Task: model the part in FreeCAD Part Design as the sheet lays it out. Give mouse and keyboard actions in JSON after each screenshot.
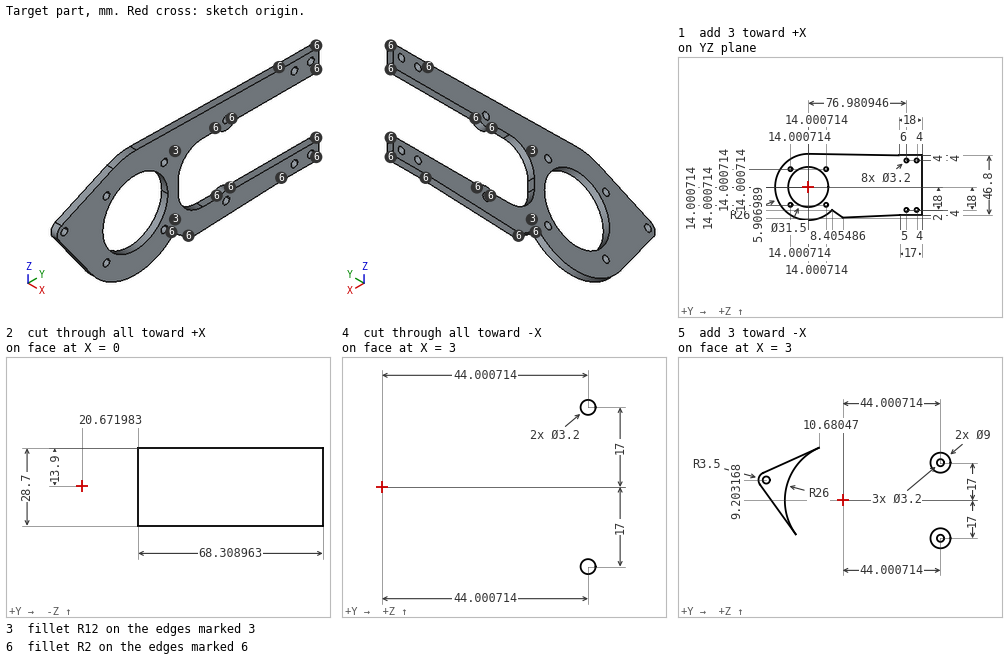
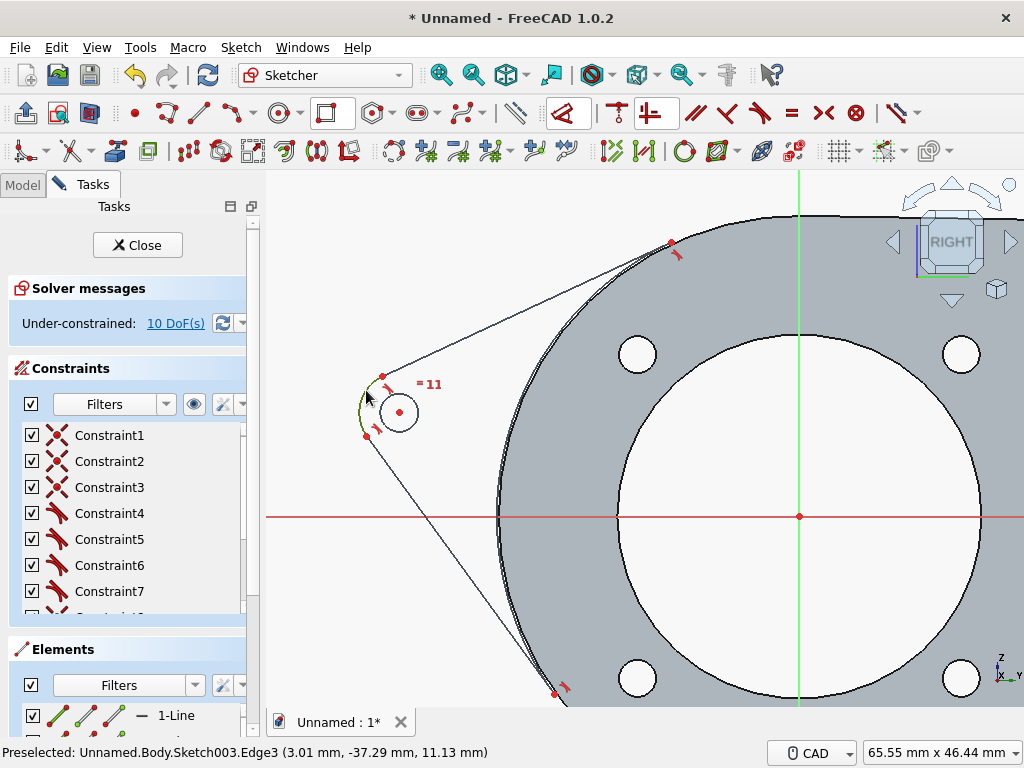
{"action": "left_click", "coordinate": [586, 114]}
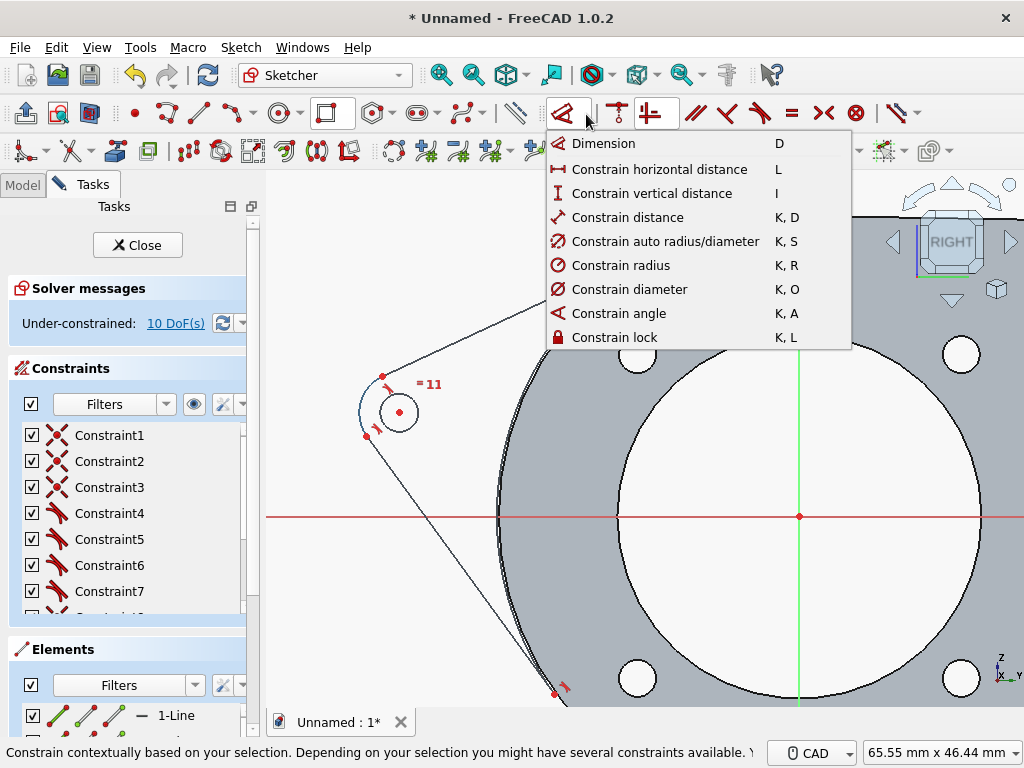
{"action": "left_click", "coordinate": [699, 265]}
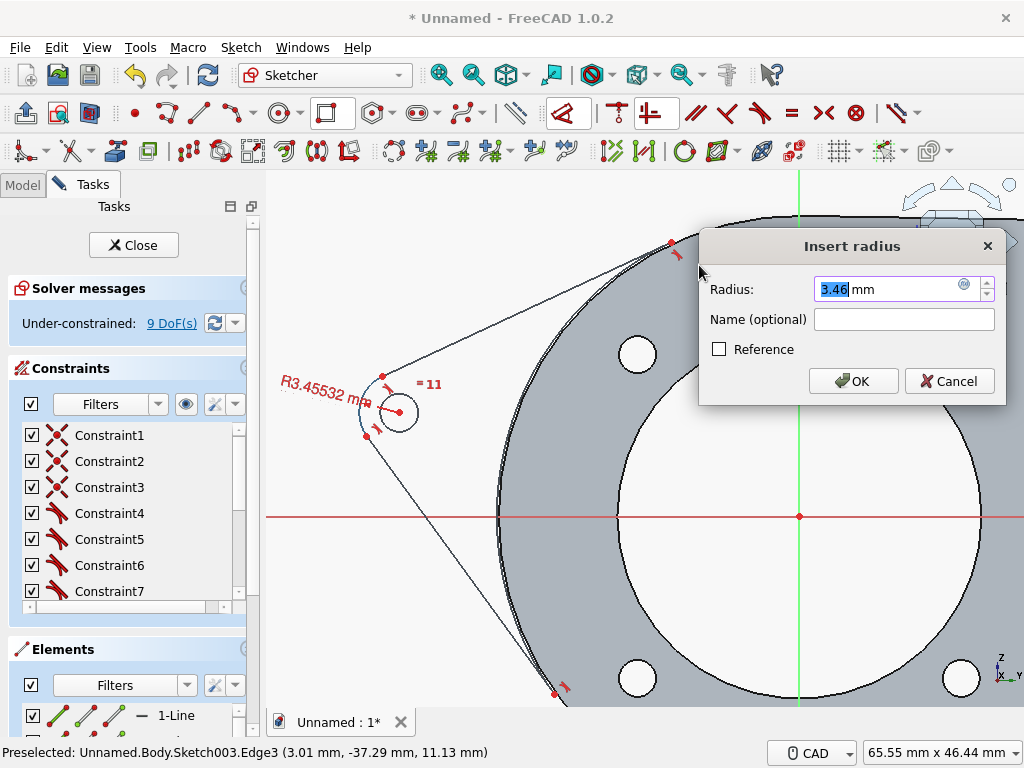
{"action": "type", "text": "3.5"}
{"action": "key", "text": "Return"}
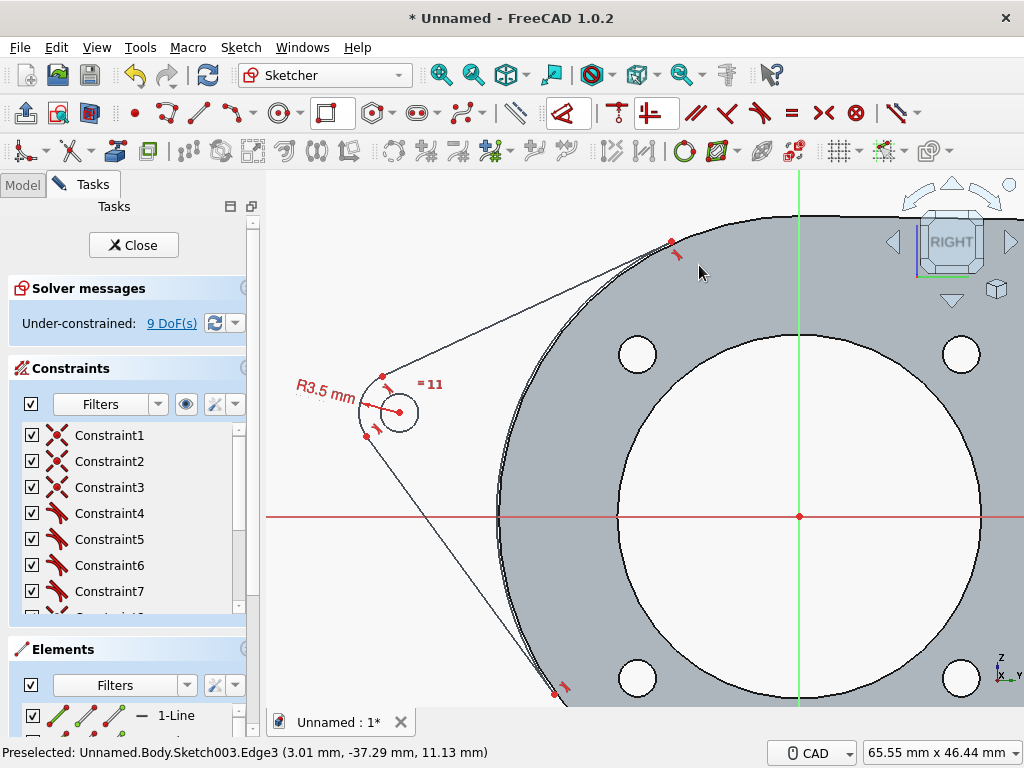
{"action": "left_click", "coordinate": [551, 344]}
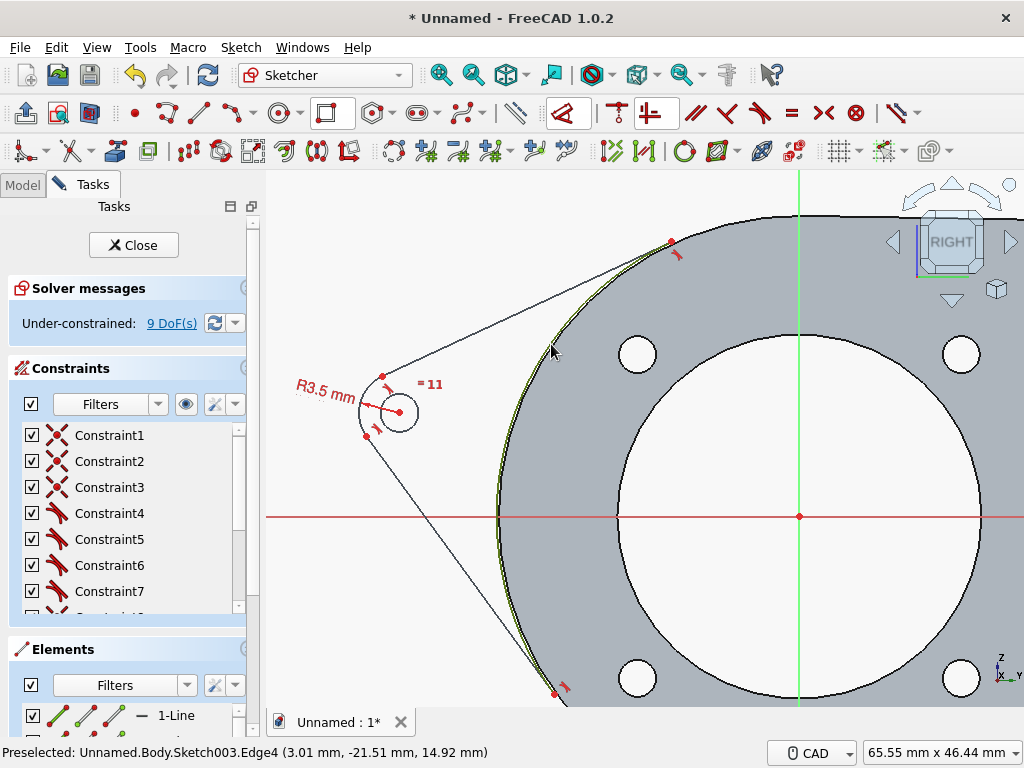
{"action": "left_click", "coordinate": [586, 114]}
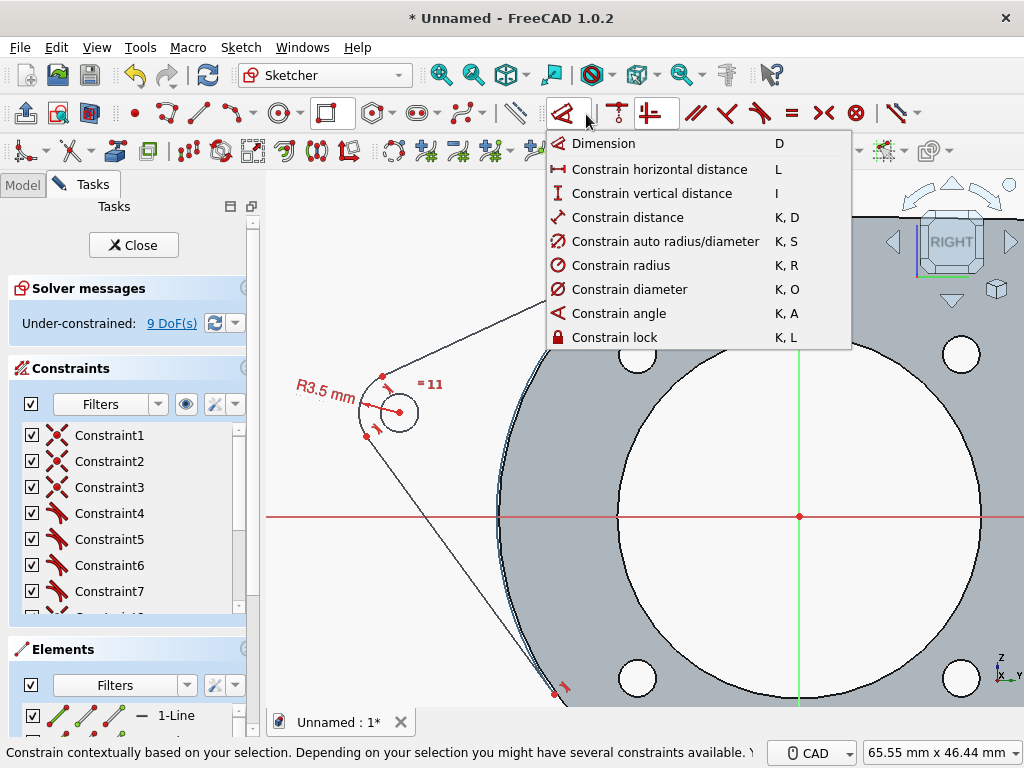
{"action": "left_click", "coordinate": [699, 265]}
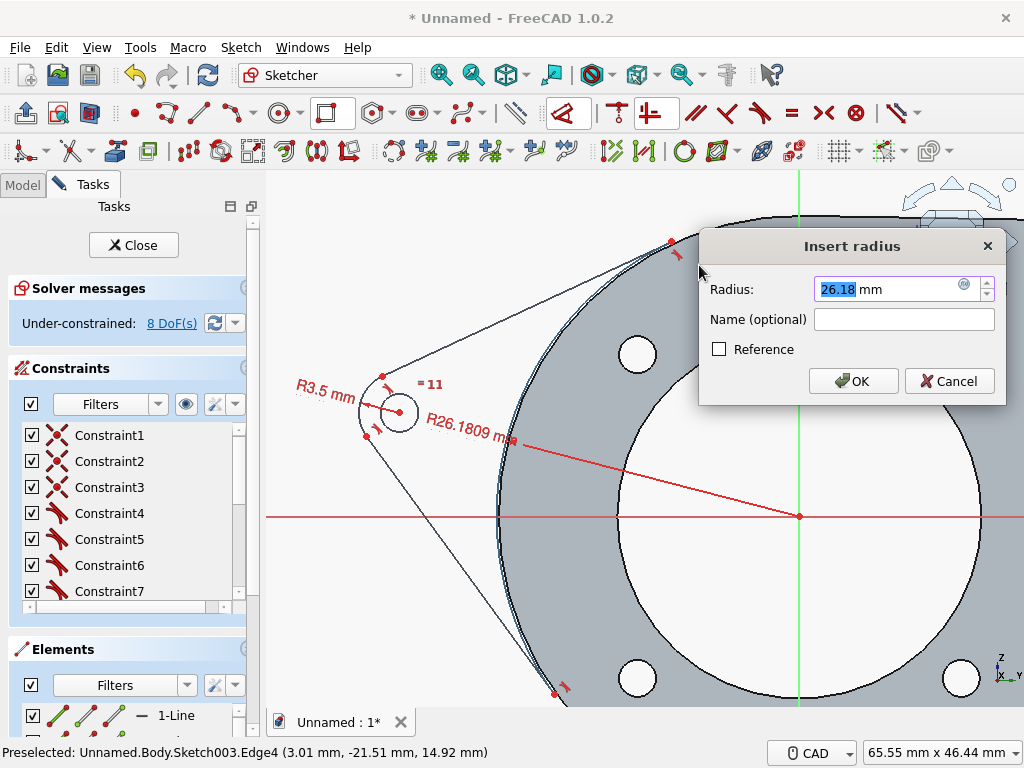
{"action": "type", "text": "26"}
{"action": "key", "text": "Return"}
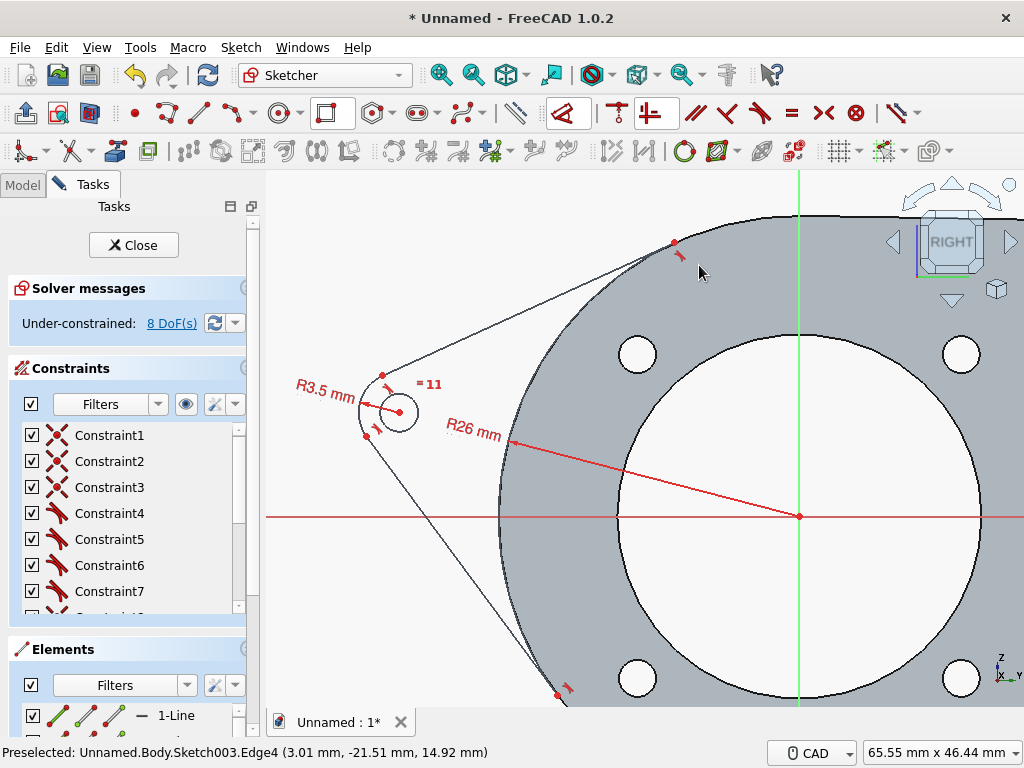
{"action": "scroll", "coordinate": [411, 401], "scroll_direction": "down", "scroll_amount": 5}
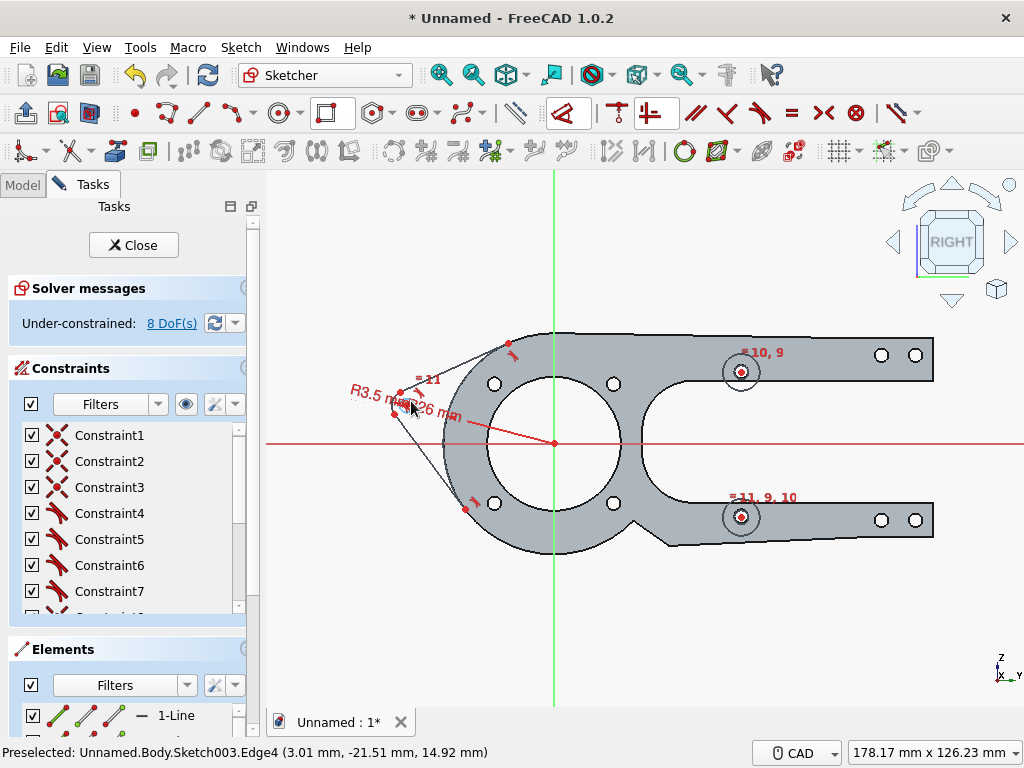
{"action": "left_click", "coordinate": [754, 359]}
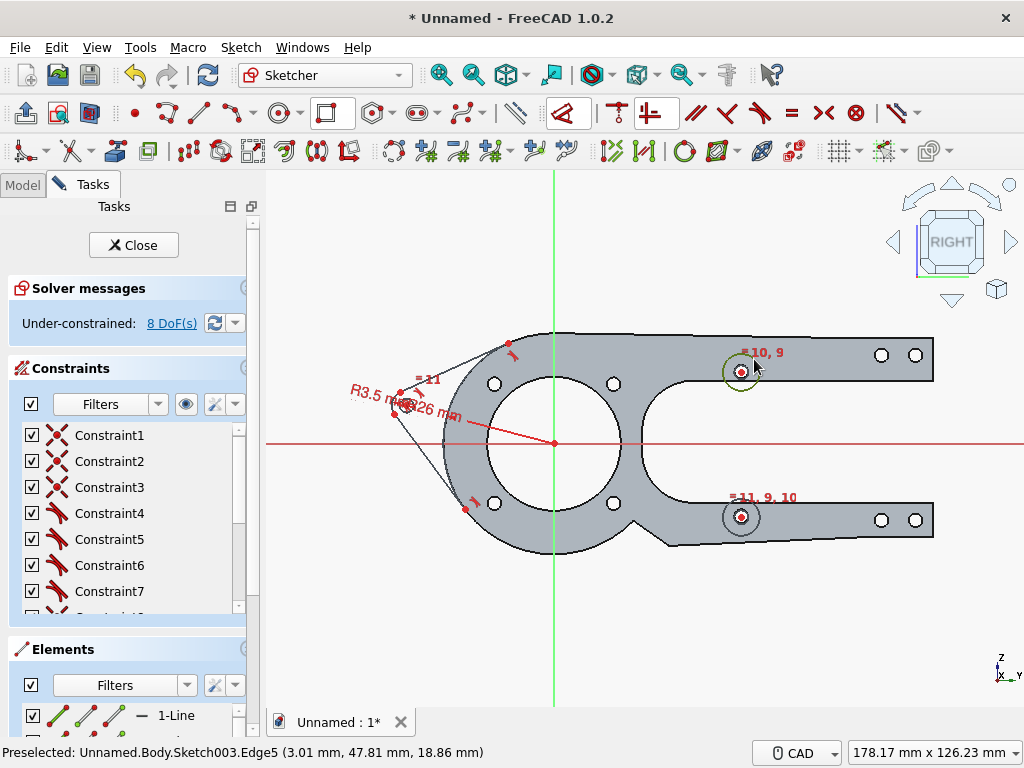
{"action": "key", "text": "k o"}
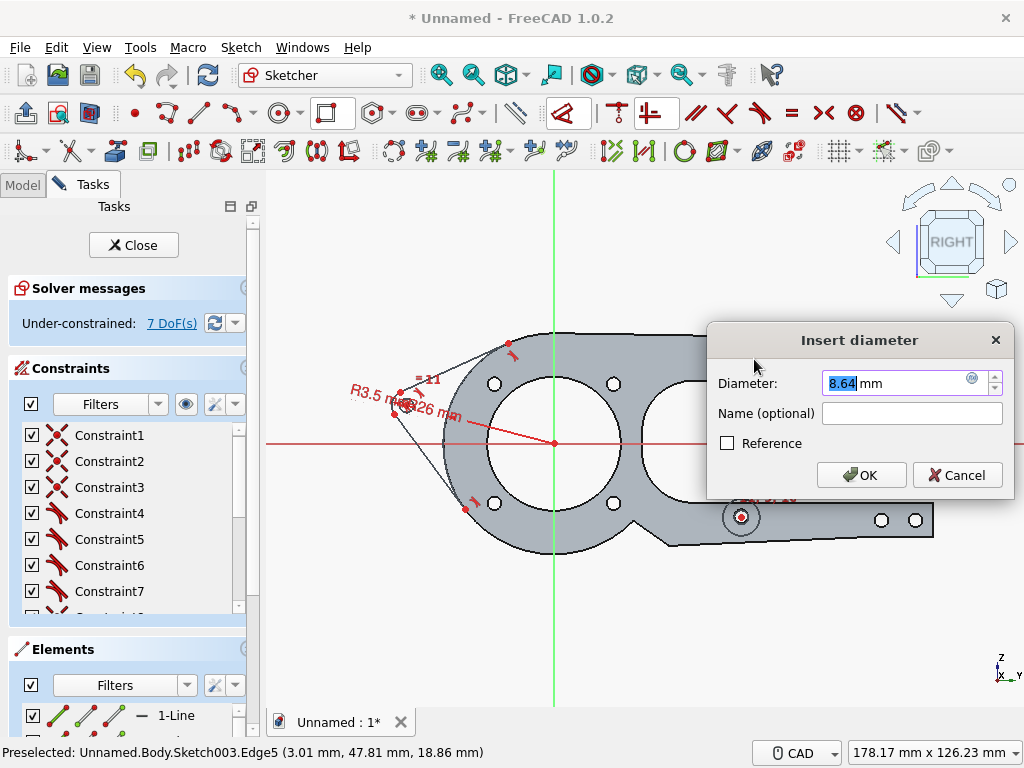
{"action": "type", "text": "9"}
{"action": "key", "text": "Return"}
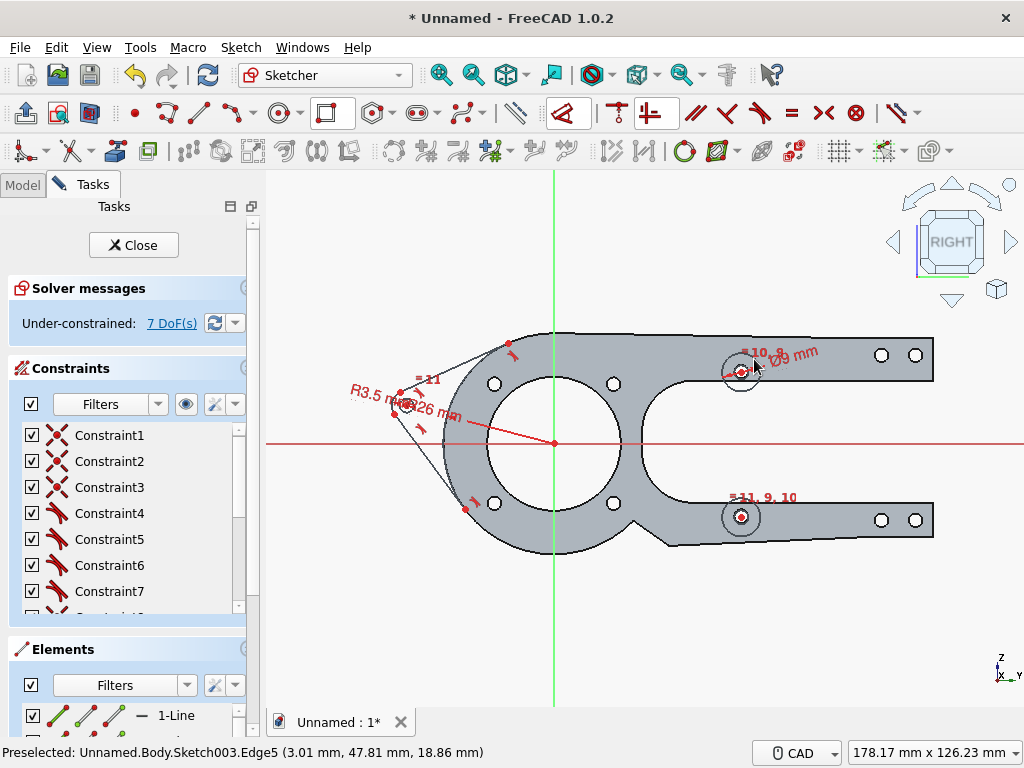
{"action": "scroll", "coordinate": [736, 367], "scroll_direction": "up", "scroll_amount": 6}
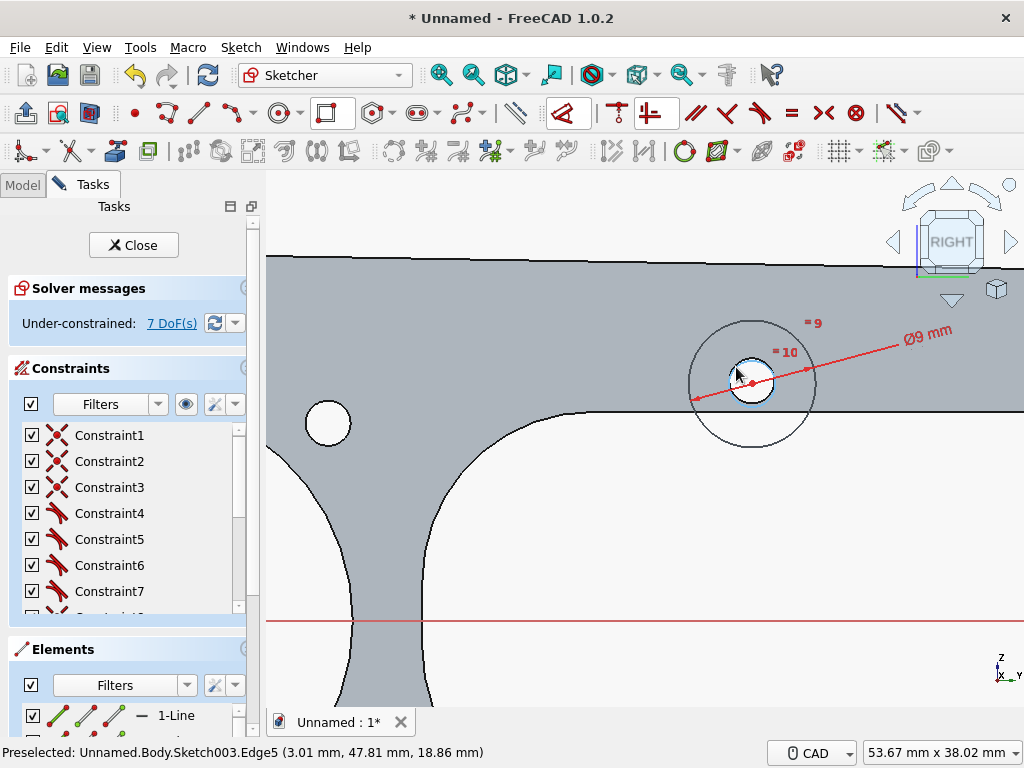
{"action": "left_click", "coordinate": [736, 368]}